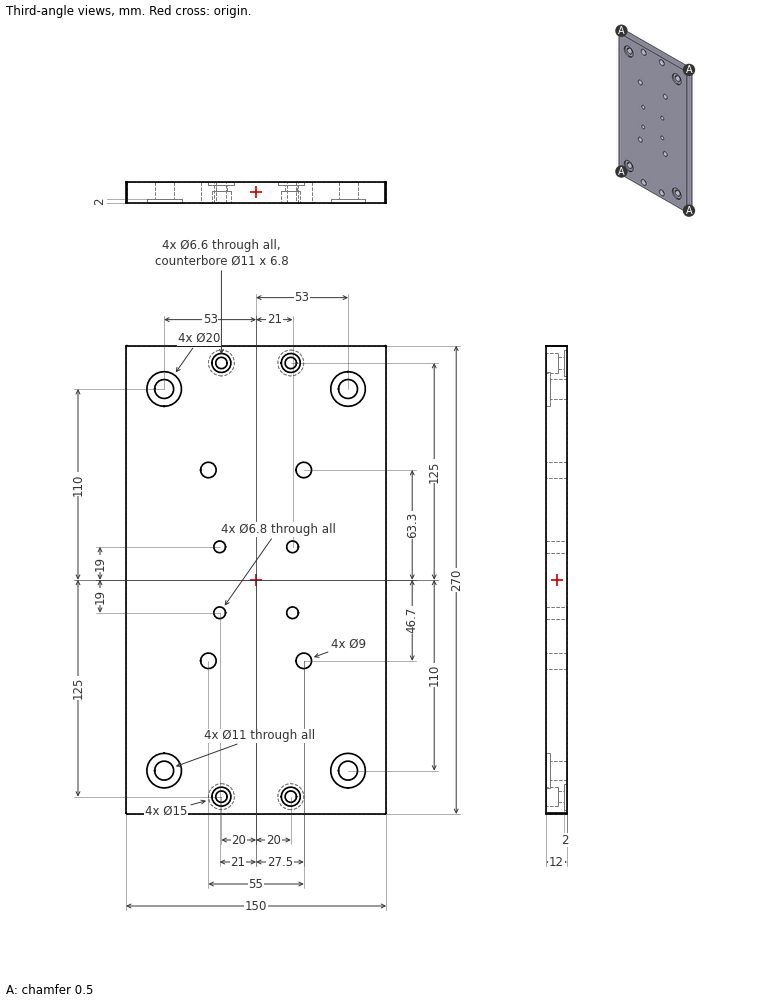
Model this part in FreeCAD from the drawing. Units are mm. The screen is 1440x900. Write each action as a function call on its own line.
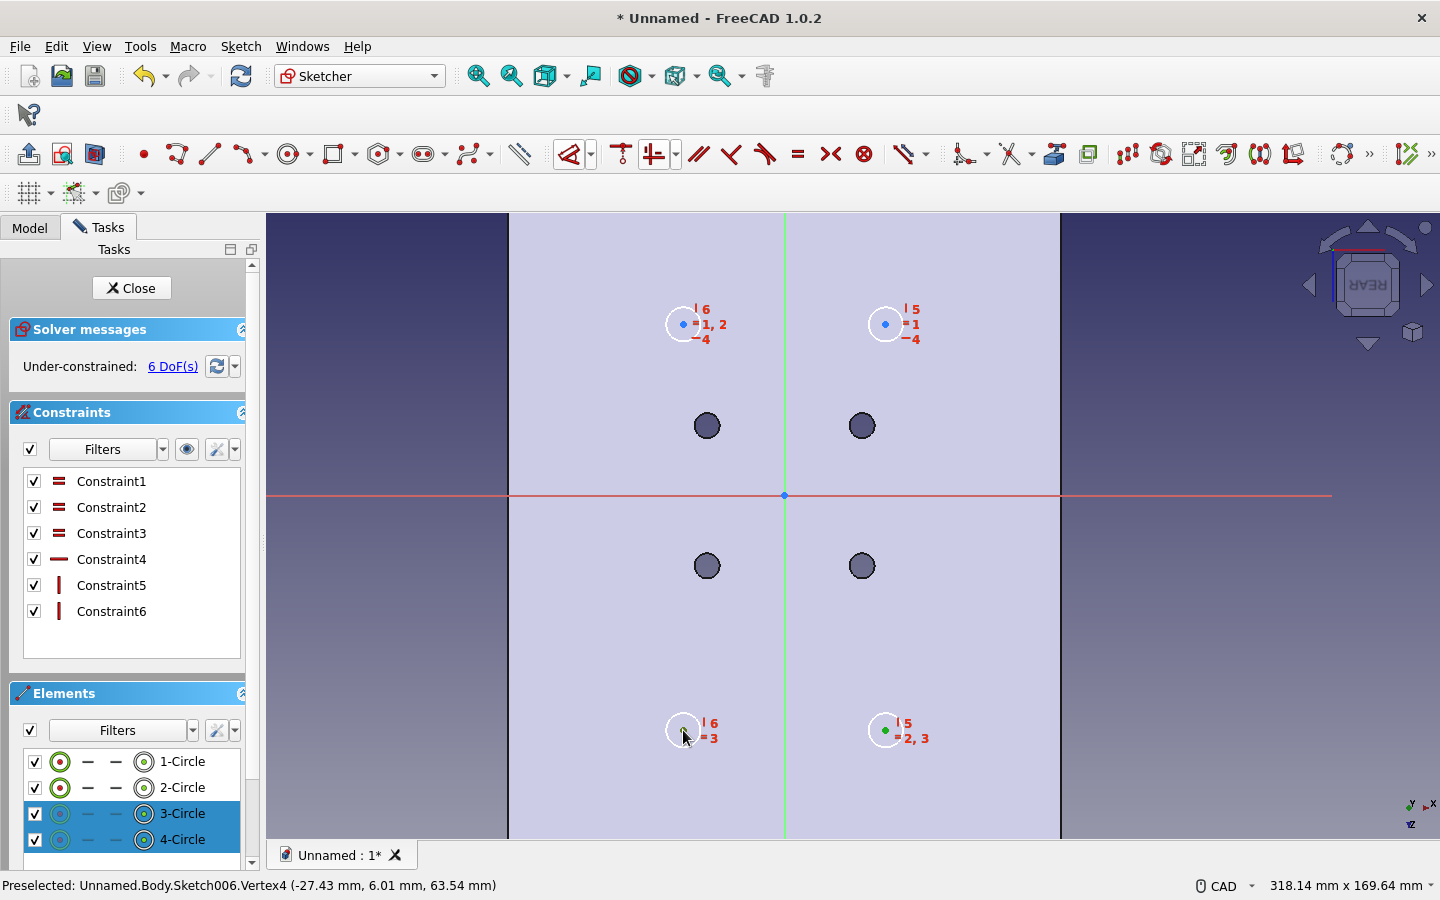
click(676, 154)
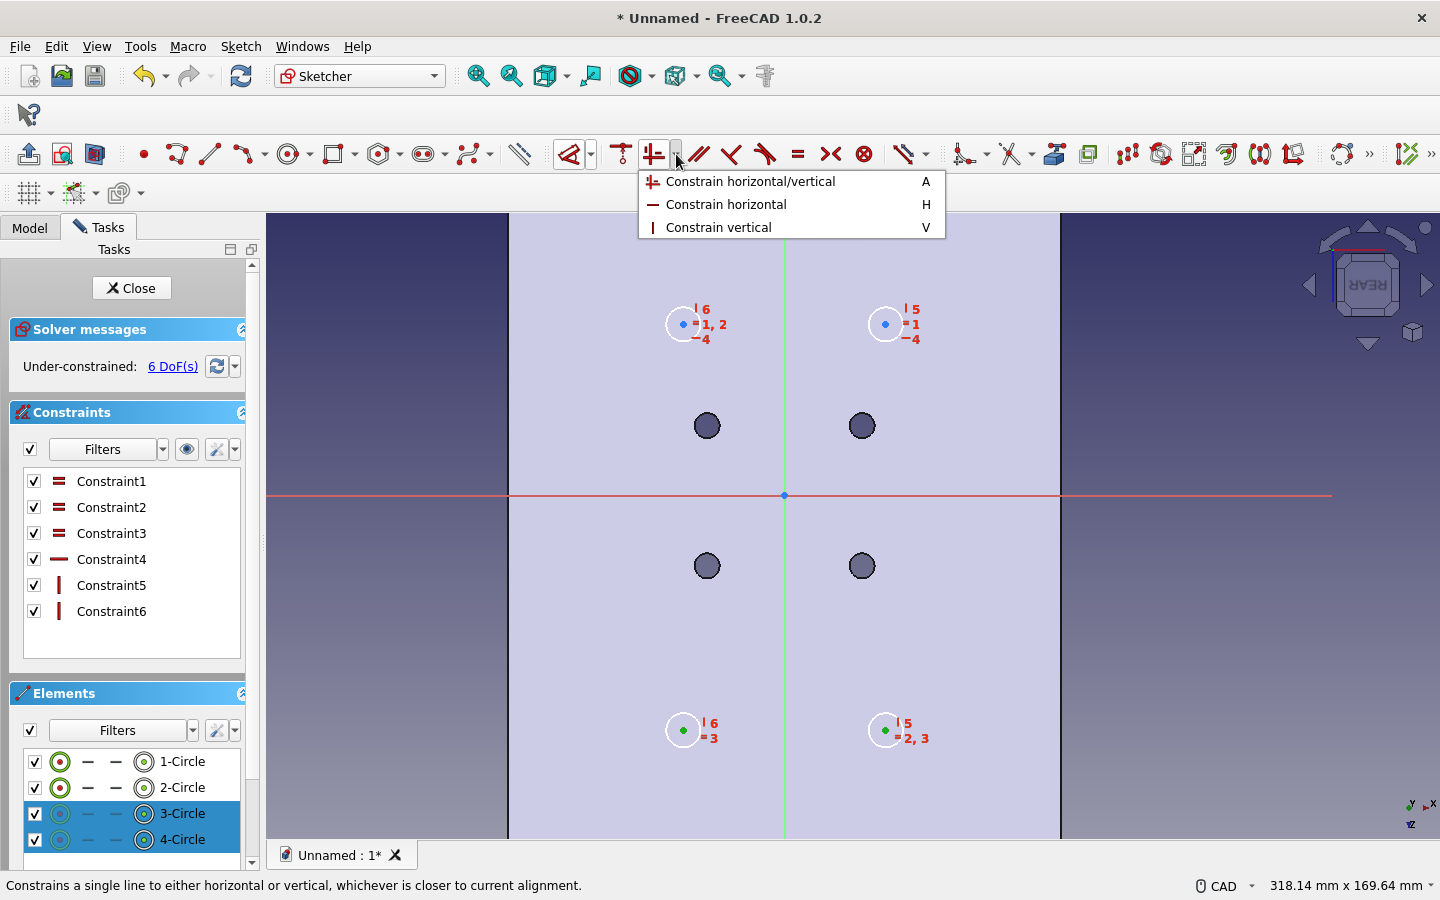
click(792, 204)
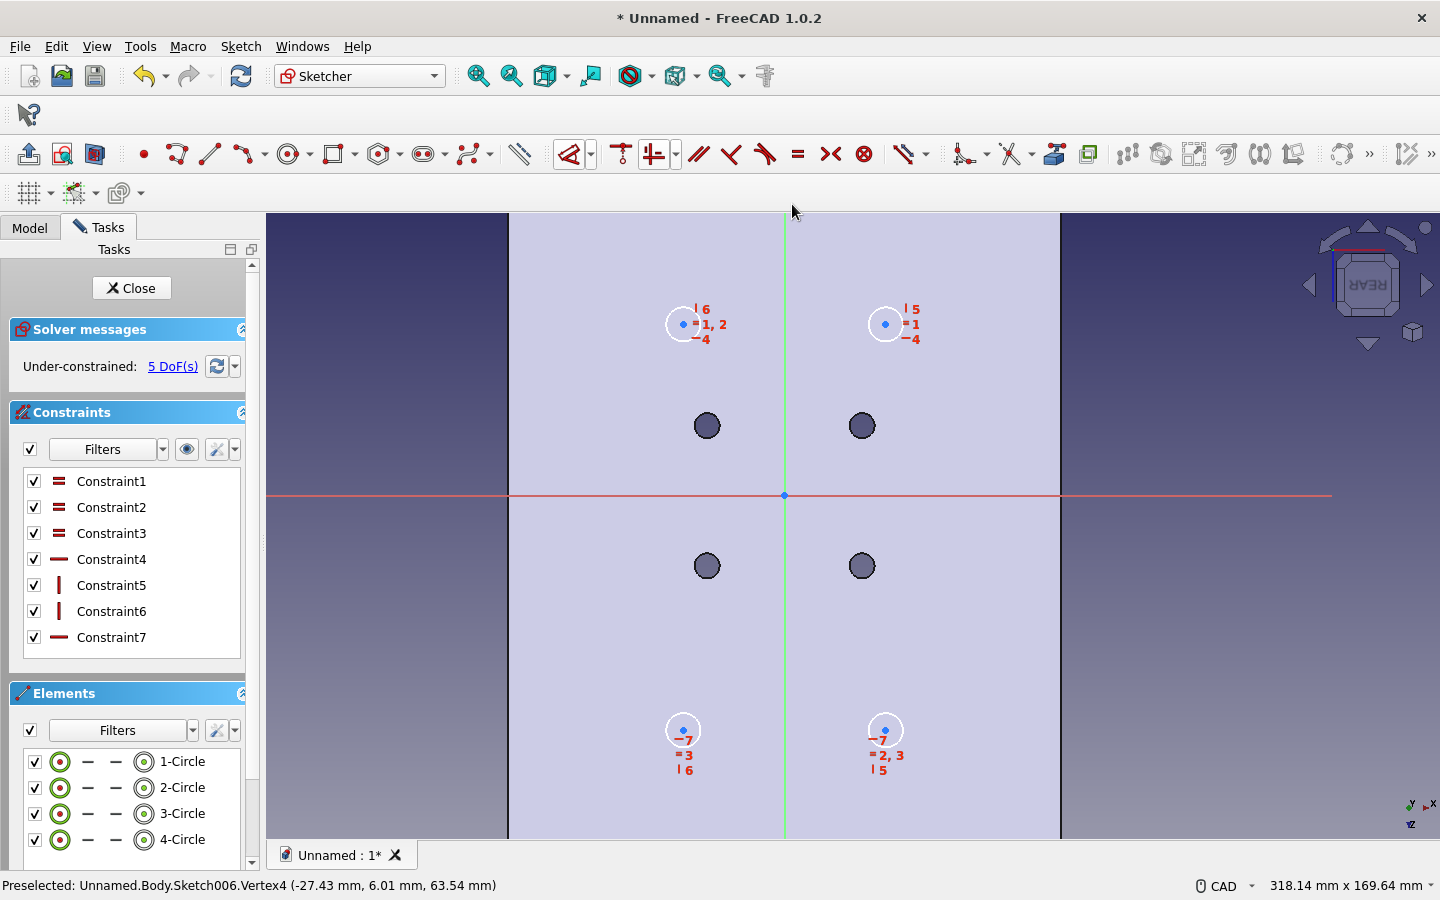
click(898, 312)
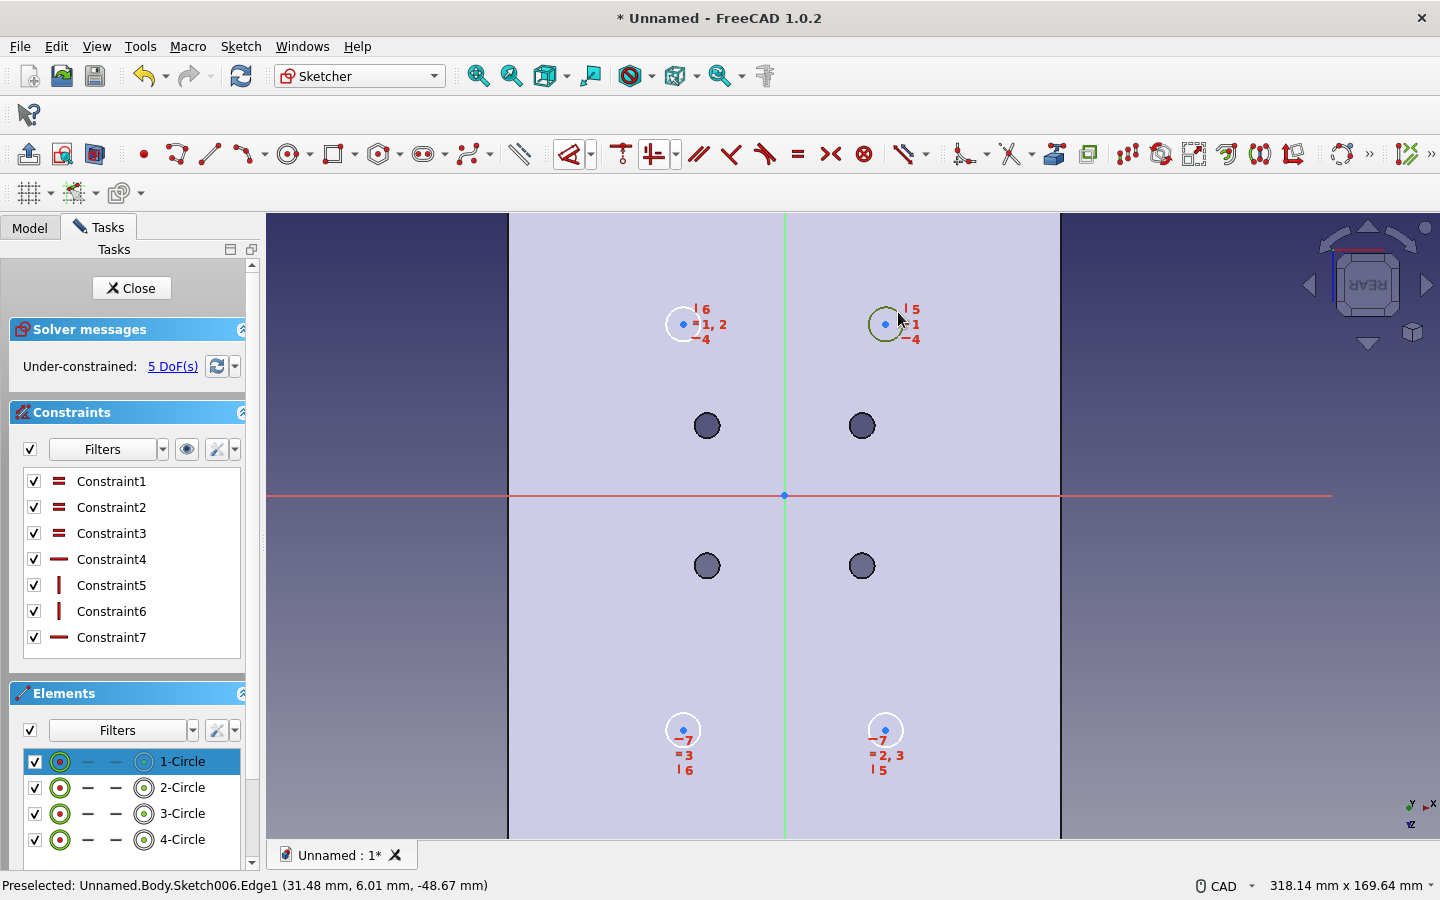
key(k)
key(o)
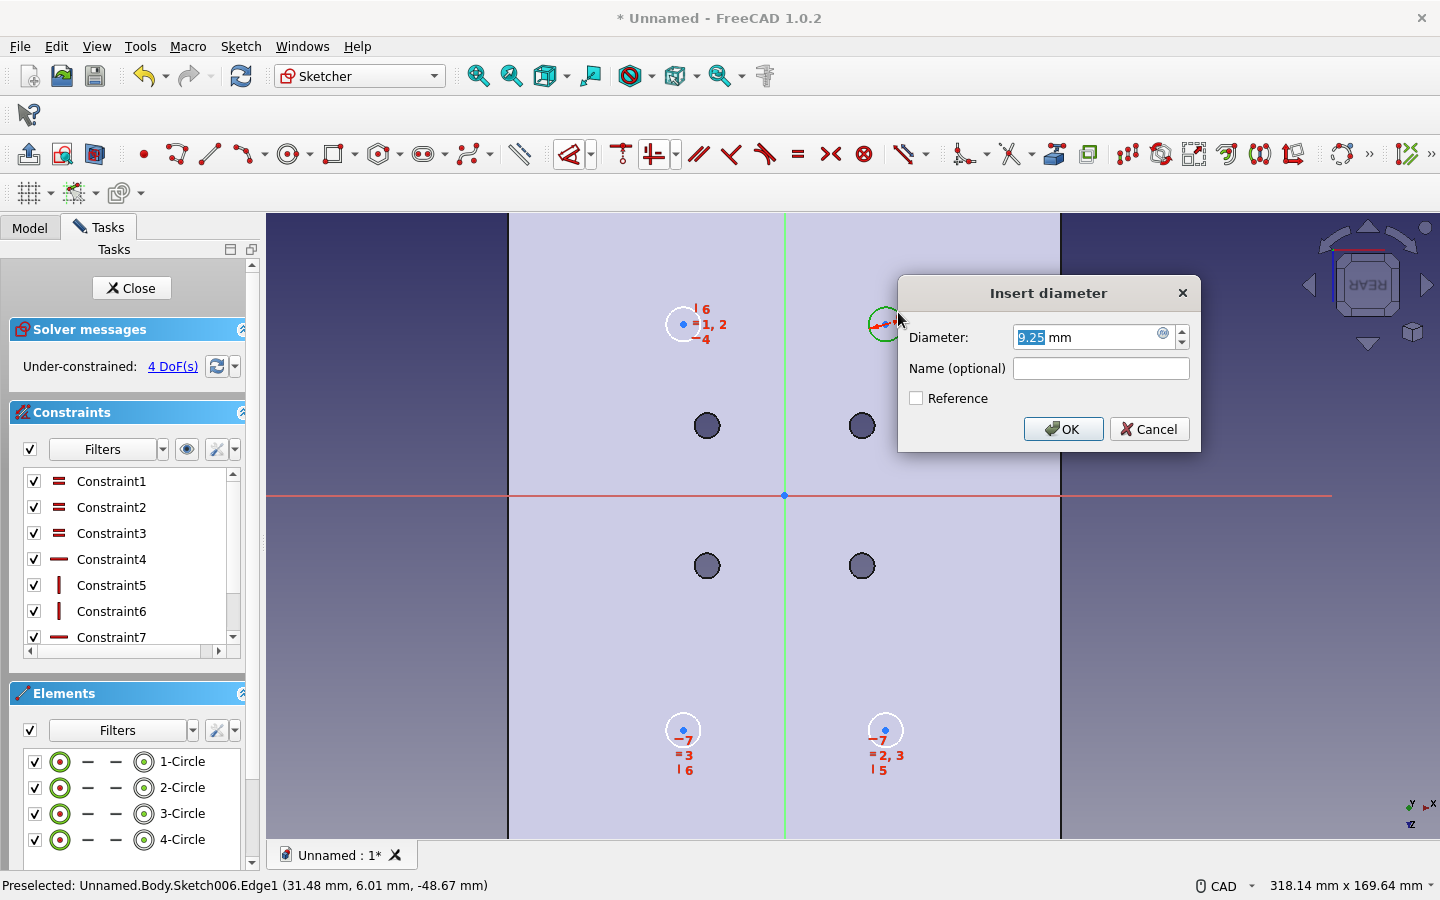
text(9)
key(Return)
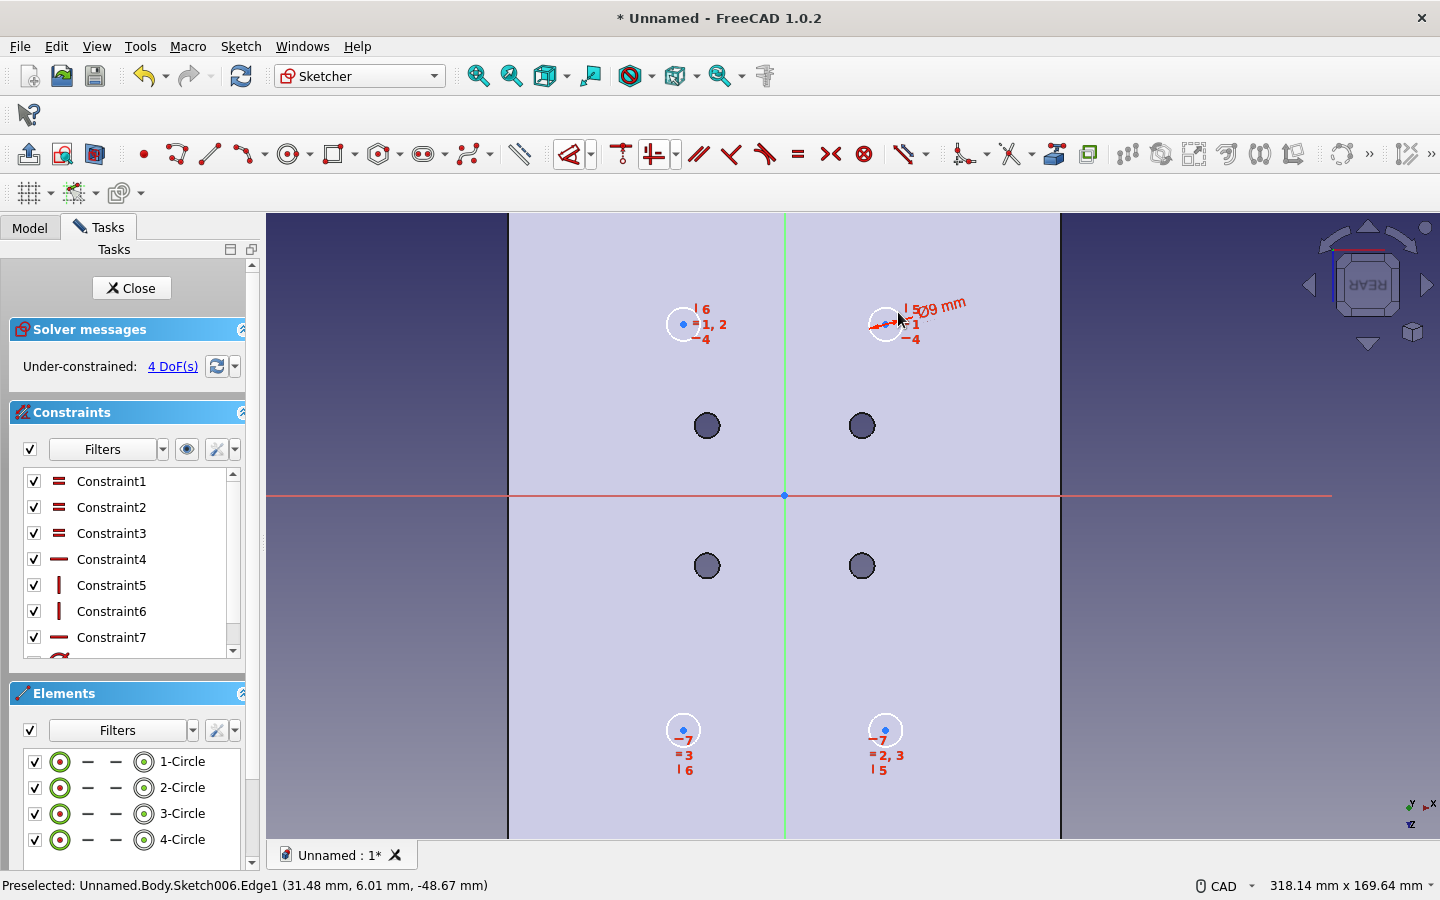
click(886, 324)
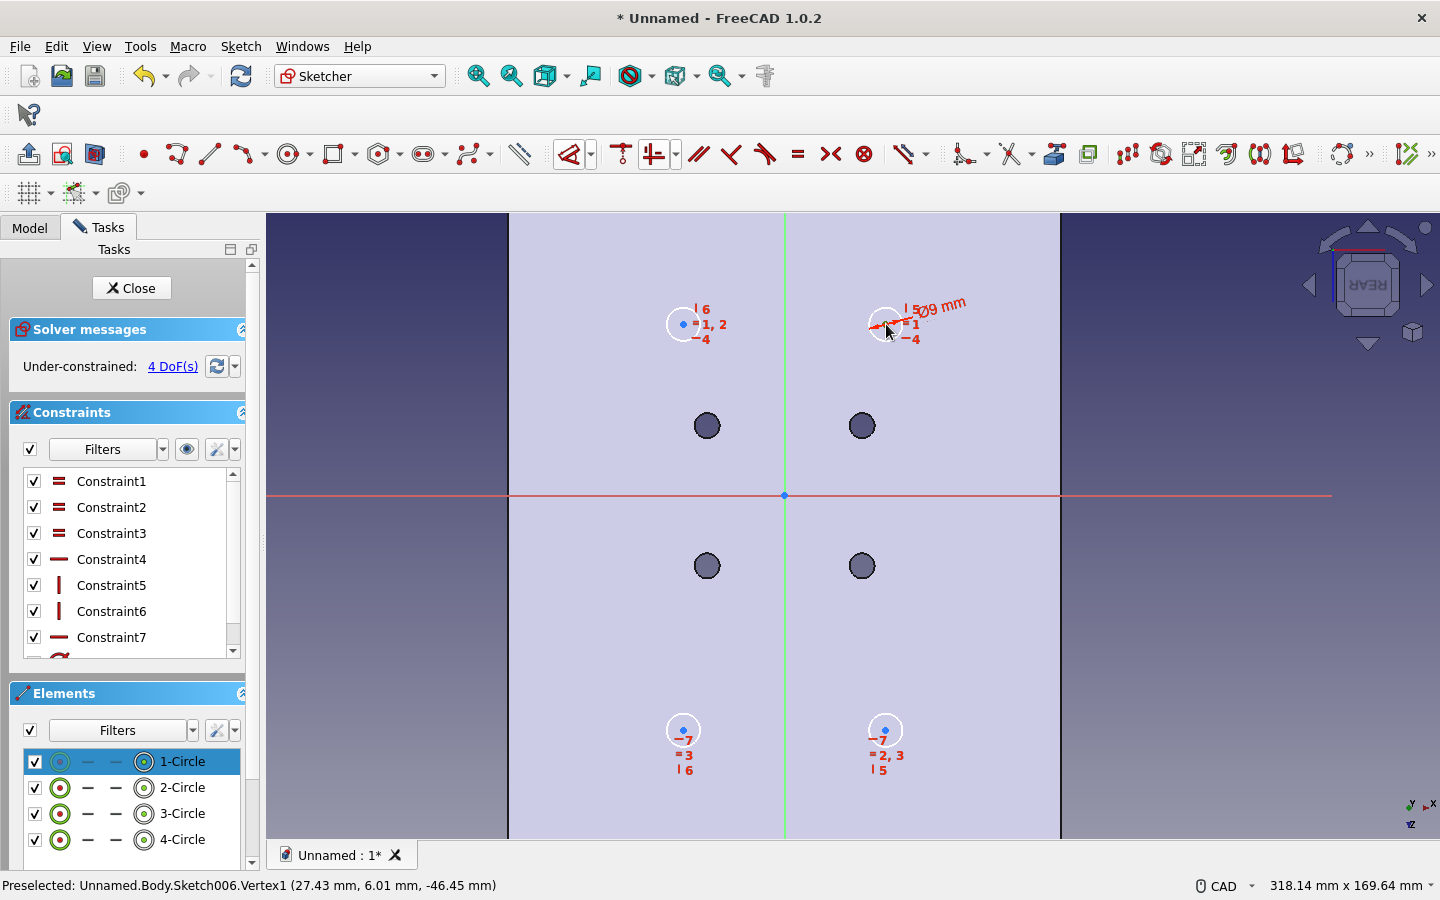
click(683, 324)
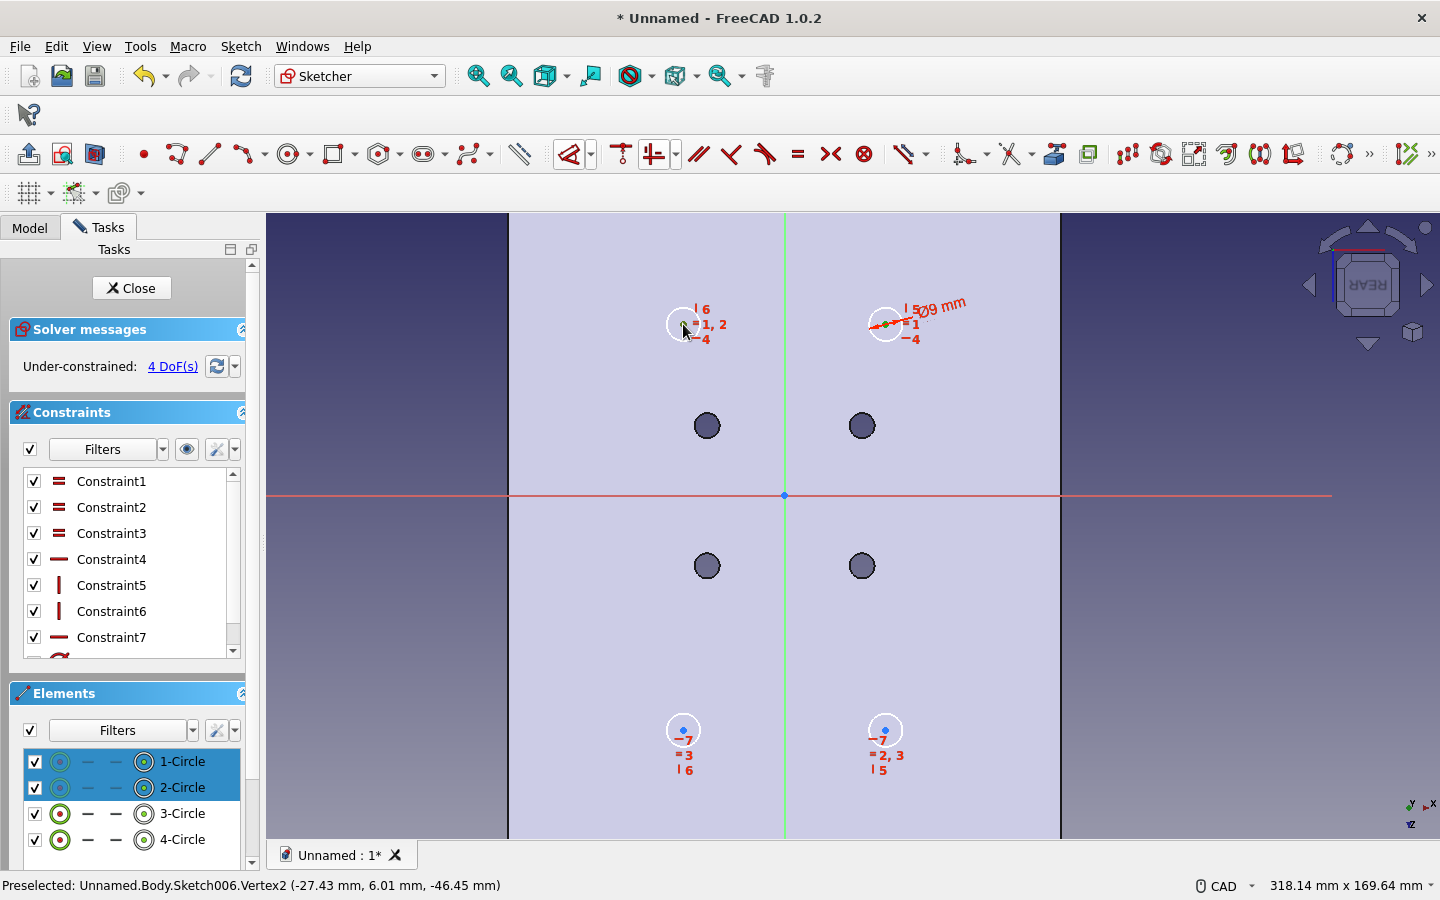
key(l)